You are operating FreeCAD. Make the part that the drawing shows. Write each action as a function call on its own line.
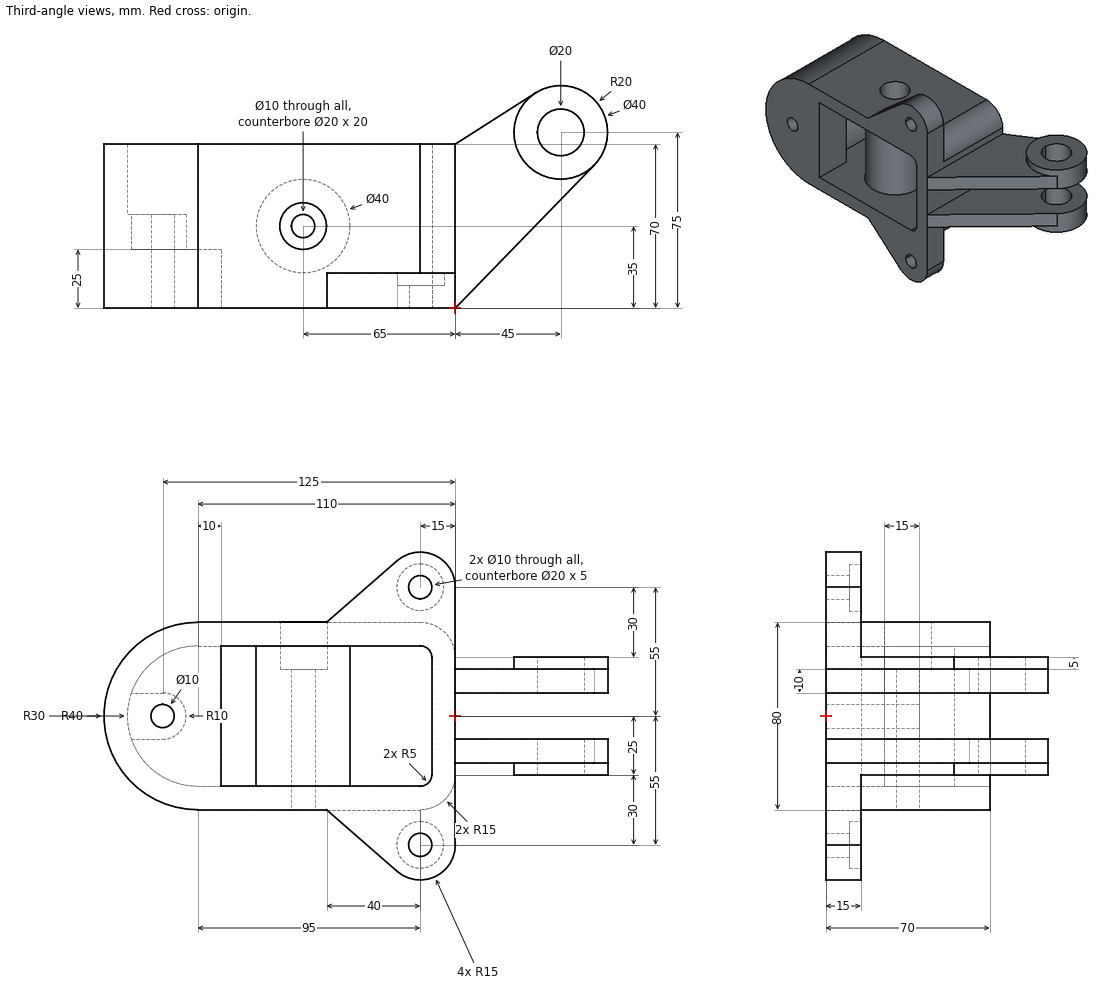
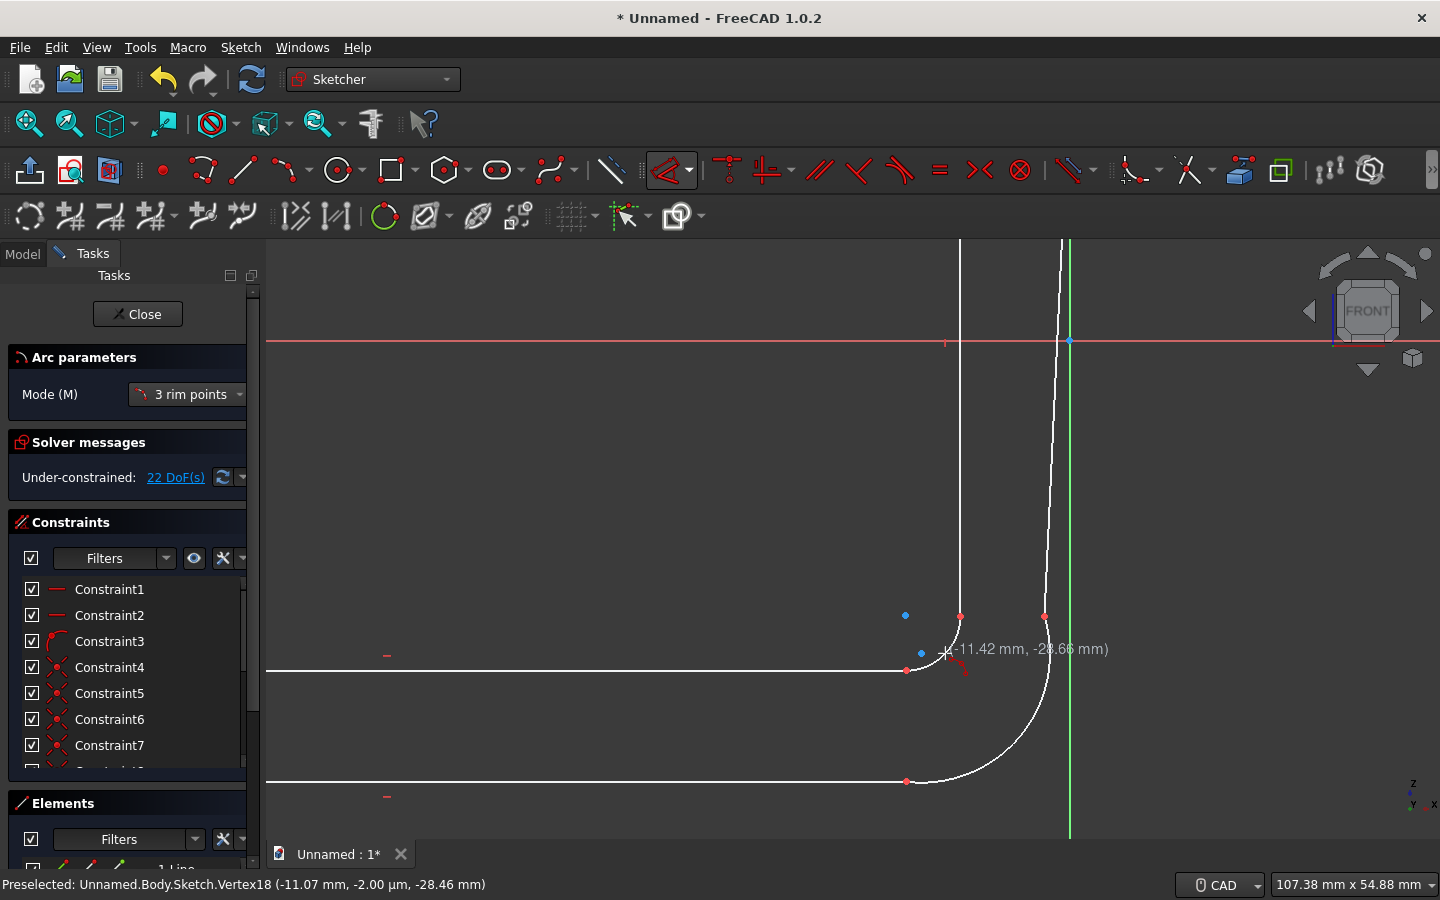
scroll(1221, 701, down, 4)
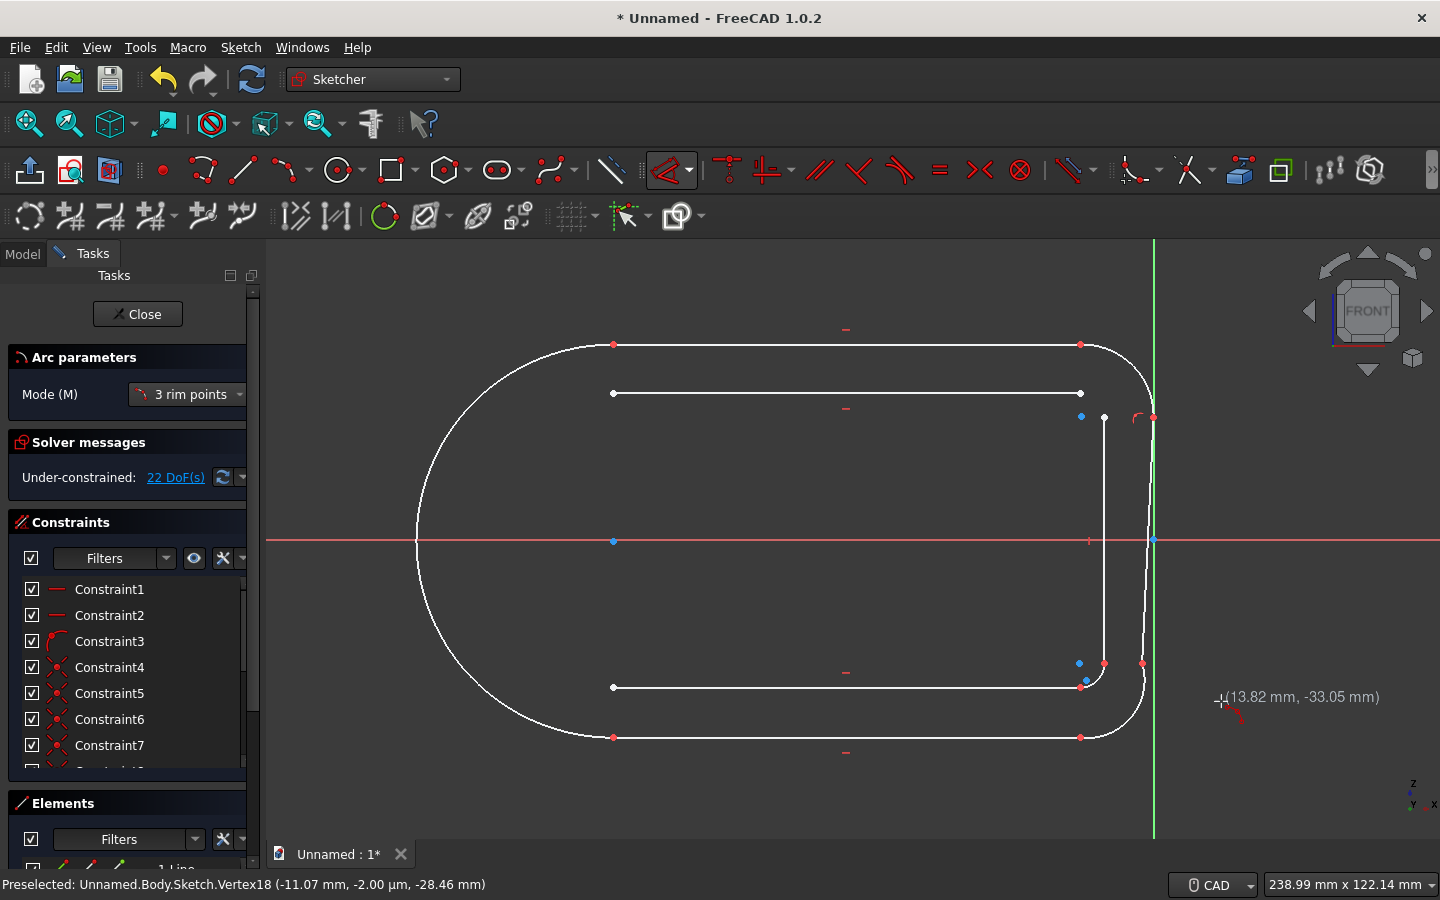
click(1104, 418)
click(1080, 393)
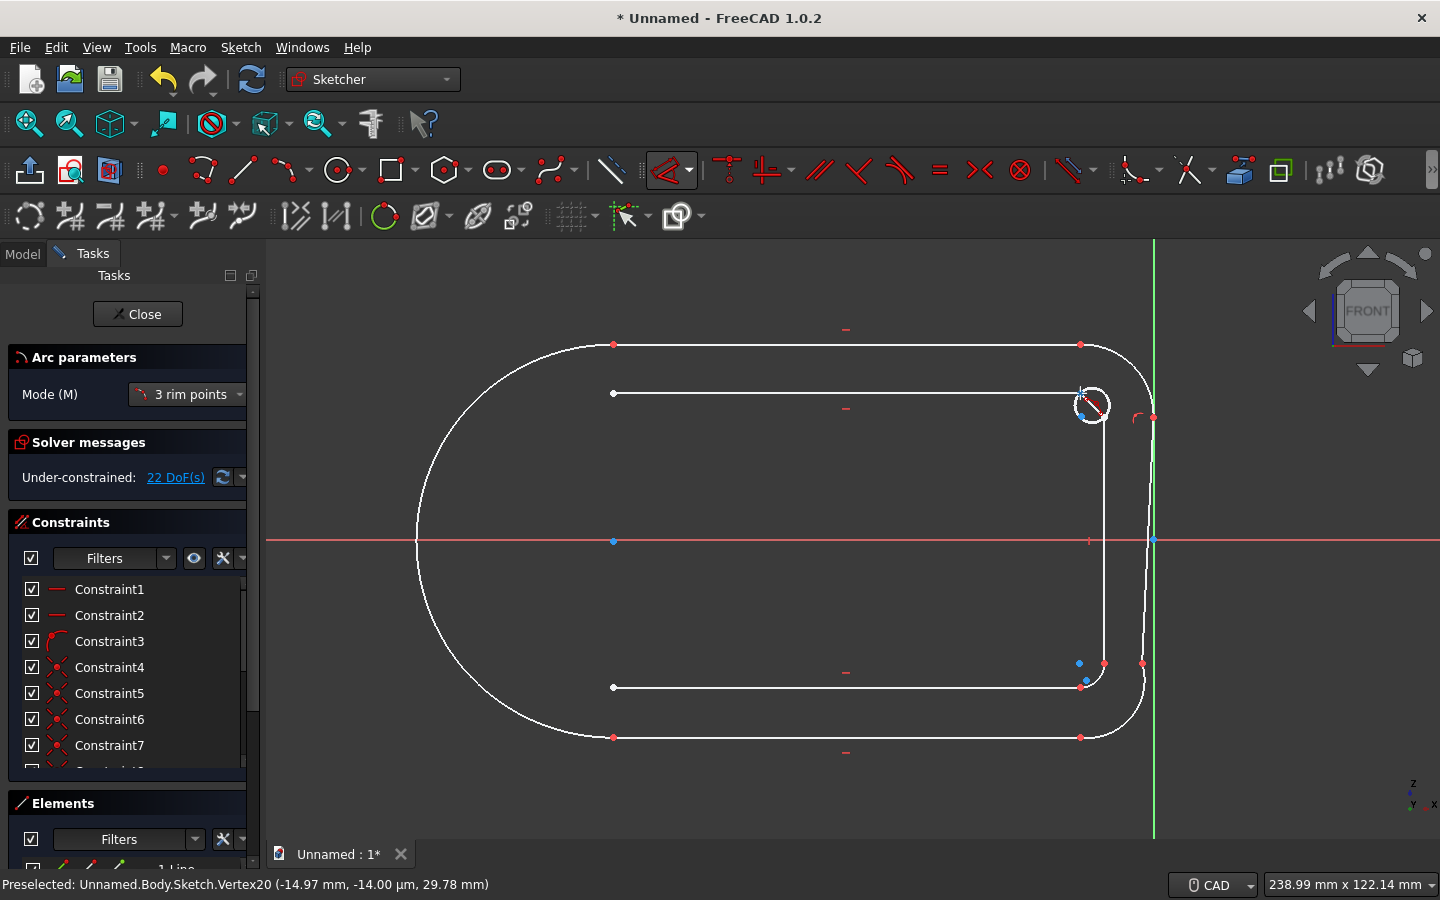
scroll(1097, 399, up, 4)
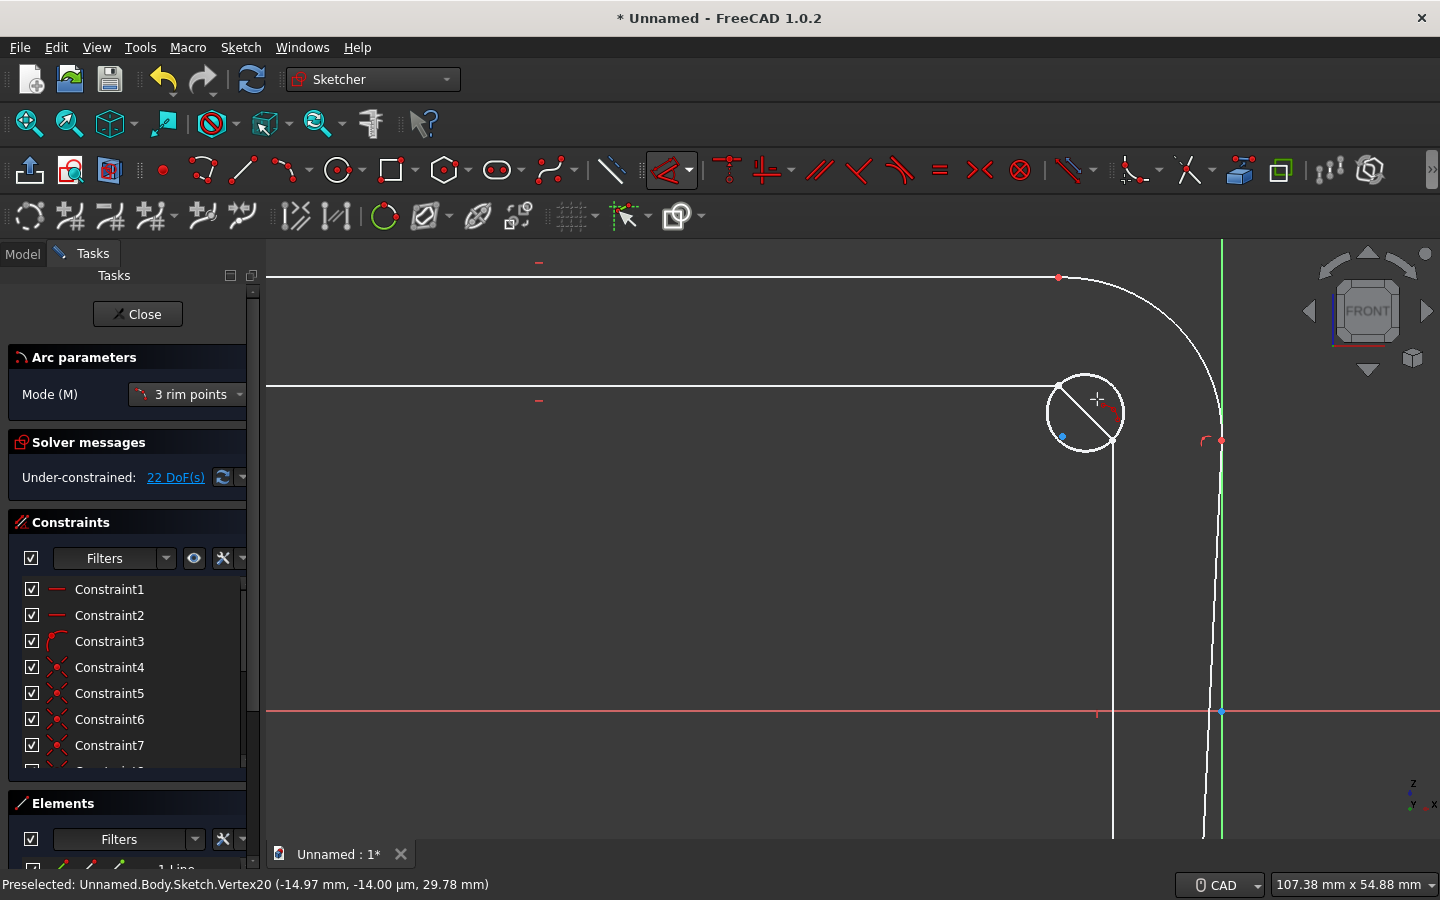
click(1097, 399)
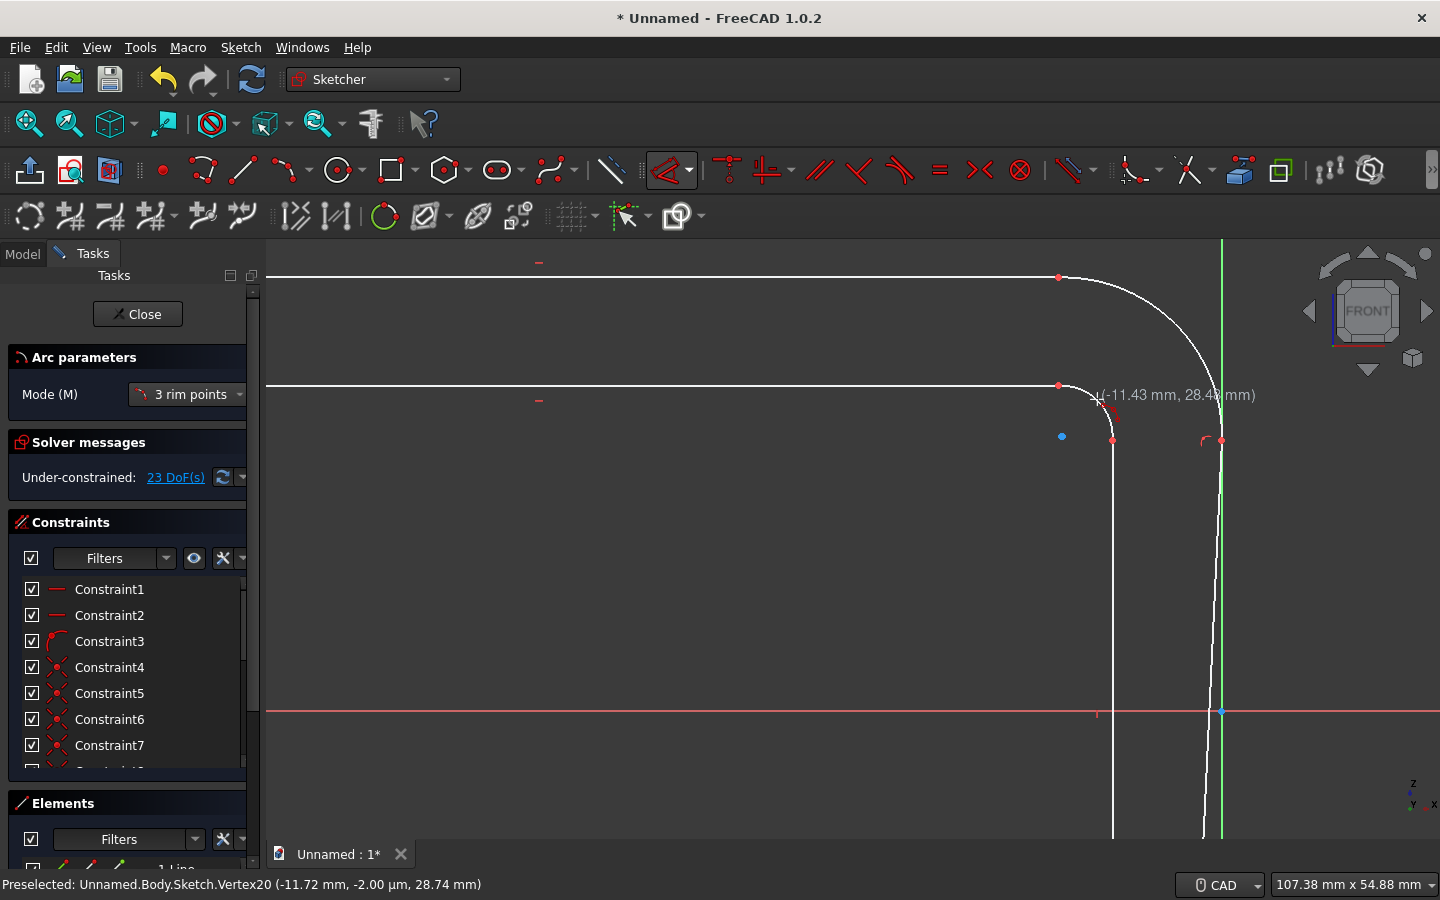
scroll(1097, 398, down, 4)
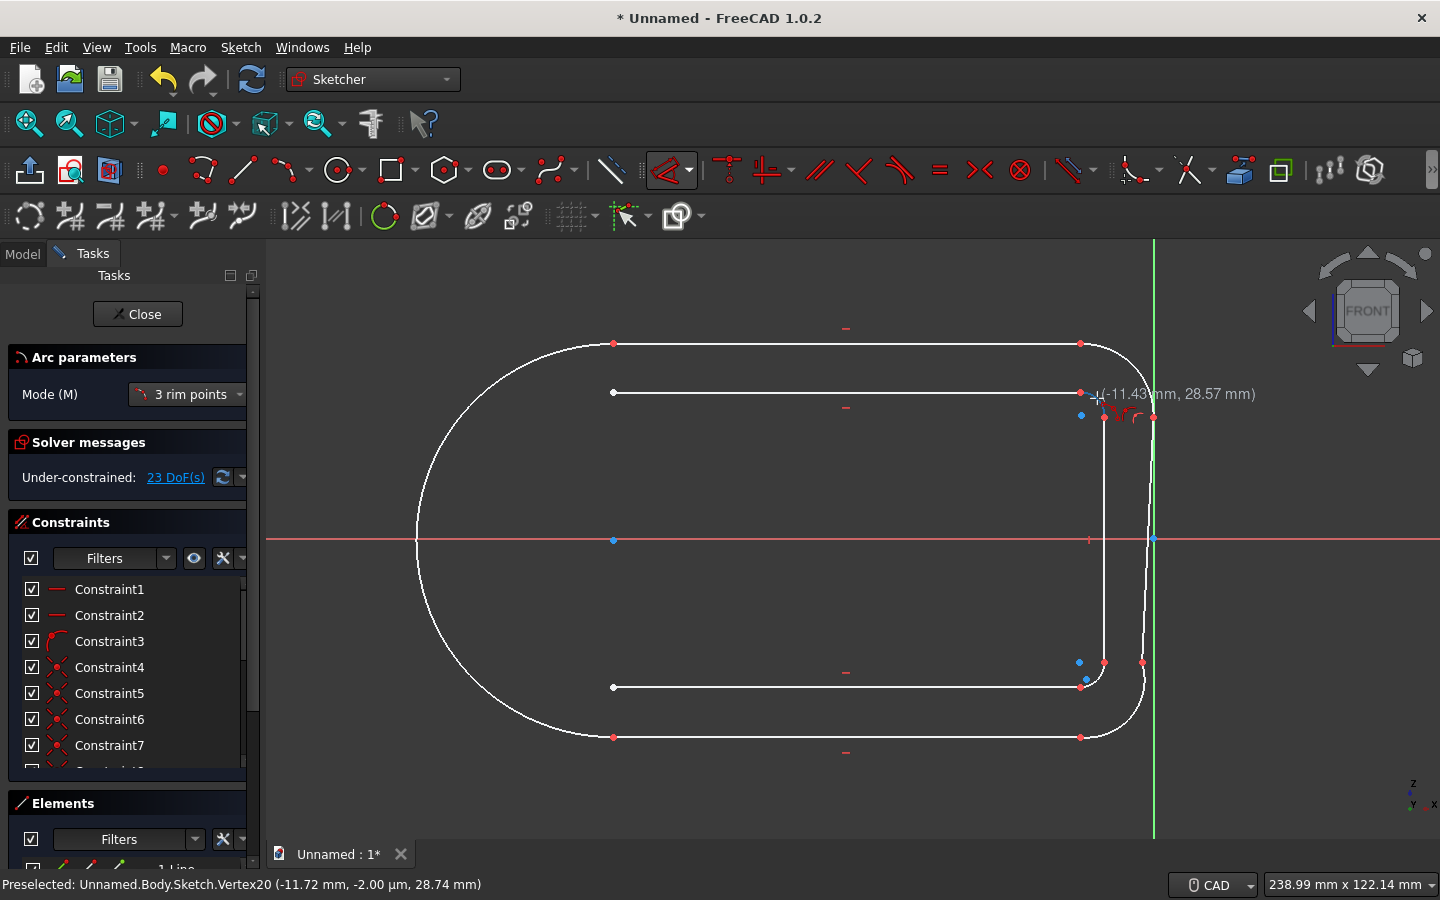
click(614, 393)
click(614, 687)
click(473, 493)
key(Escape)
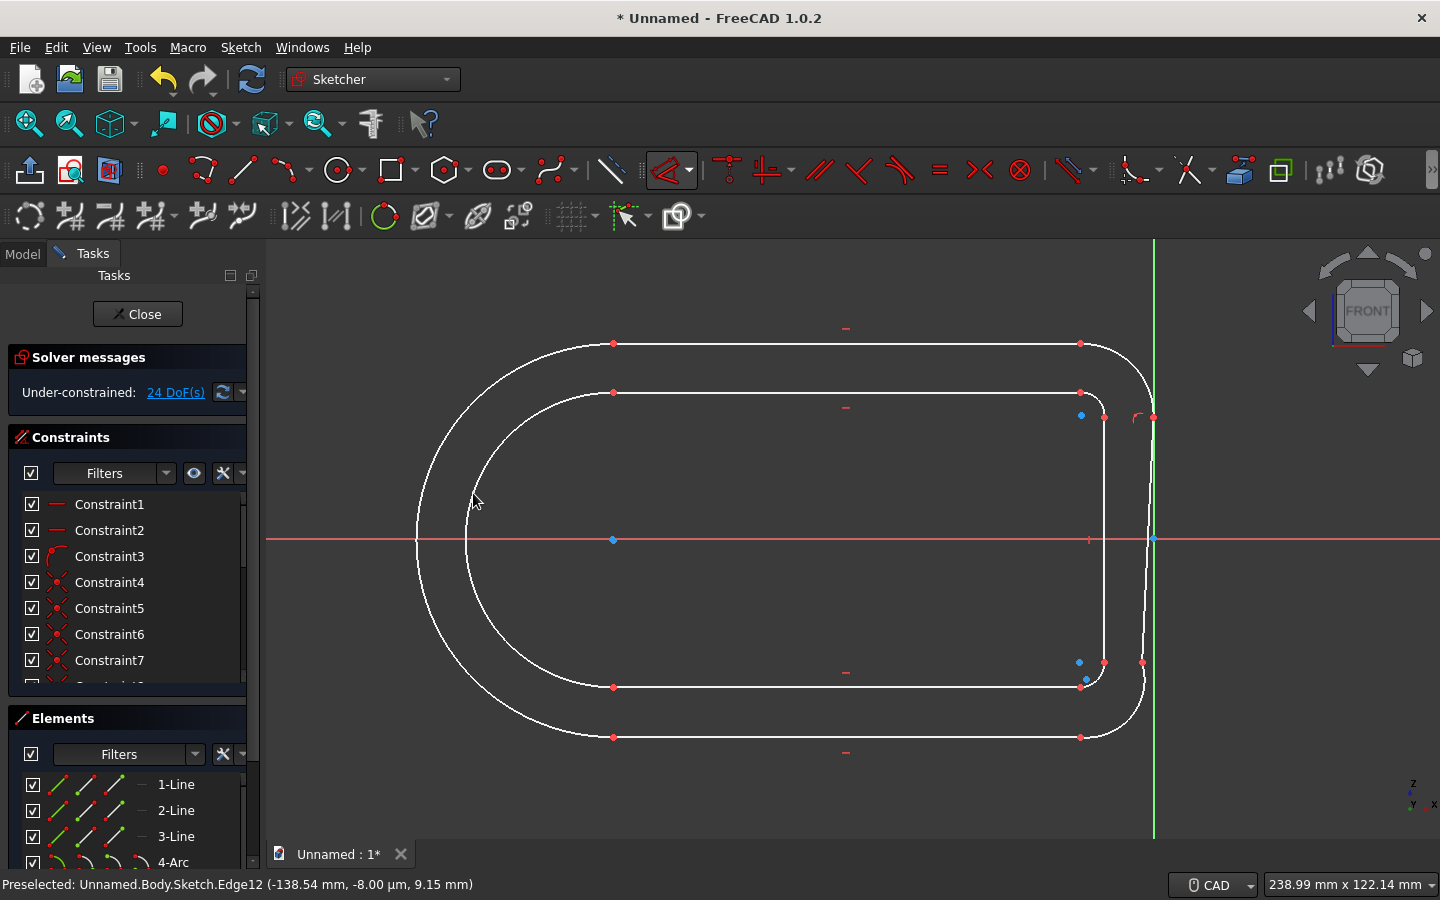
click(940, 737)